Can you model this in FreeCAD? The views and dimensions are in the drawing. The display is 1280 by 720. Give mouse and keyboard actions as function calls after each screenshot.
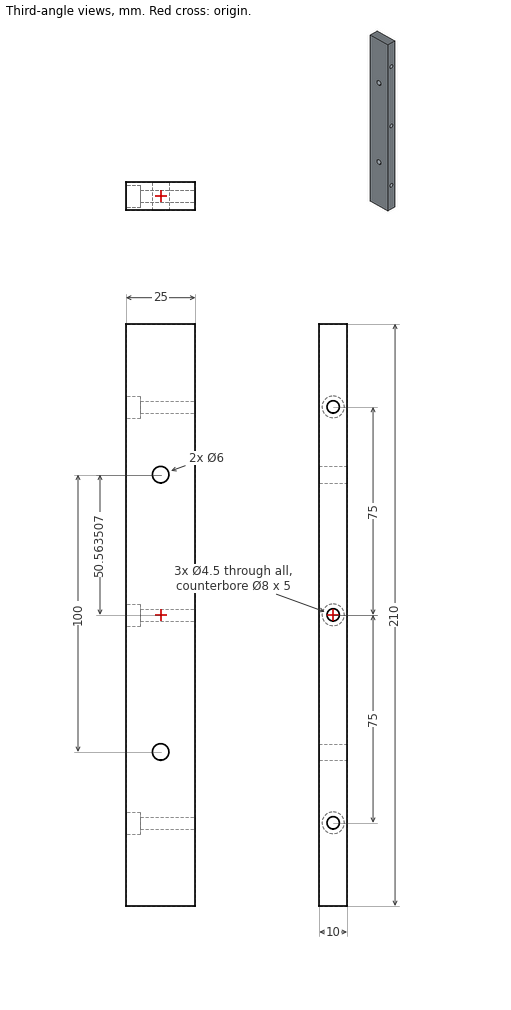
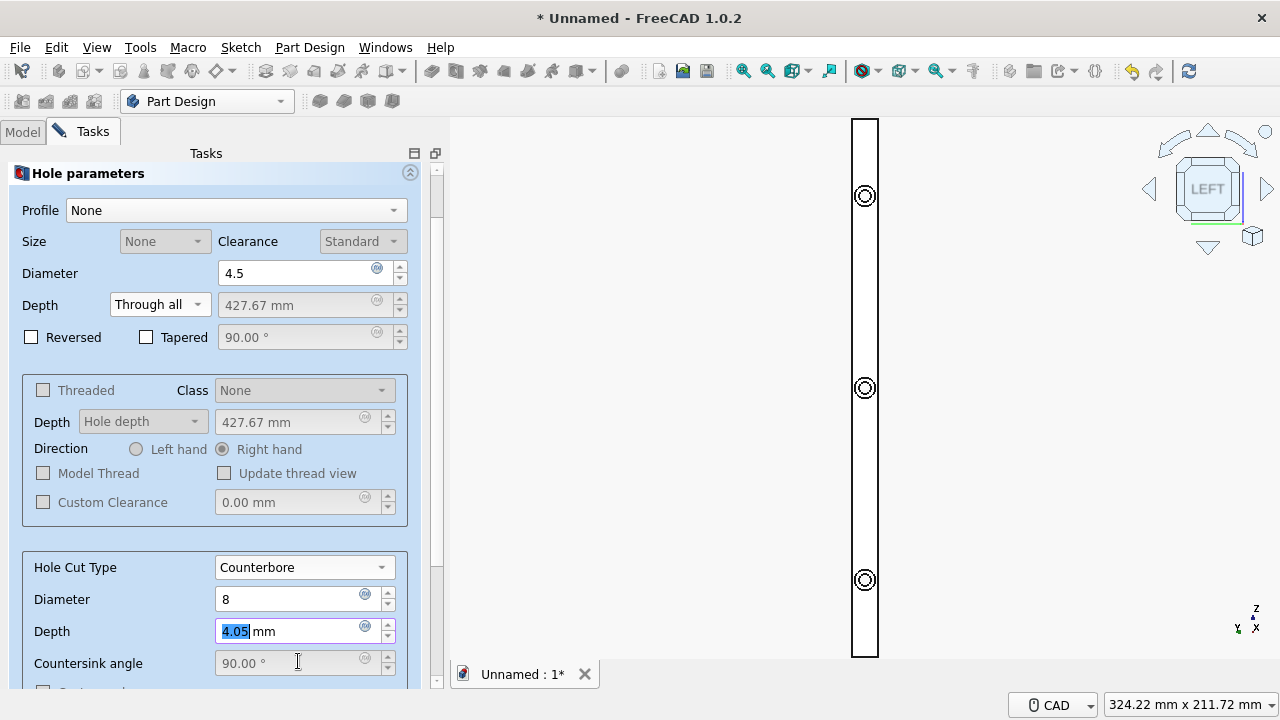
text(5)
key(Tab)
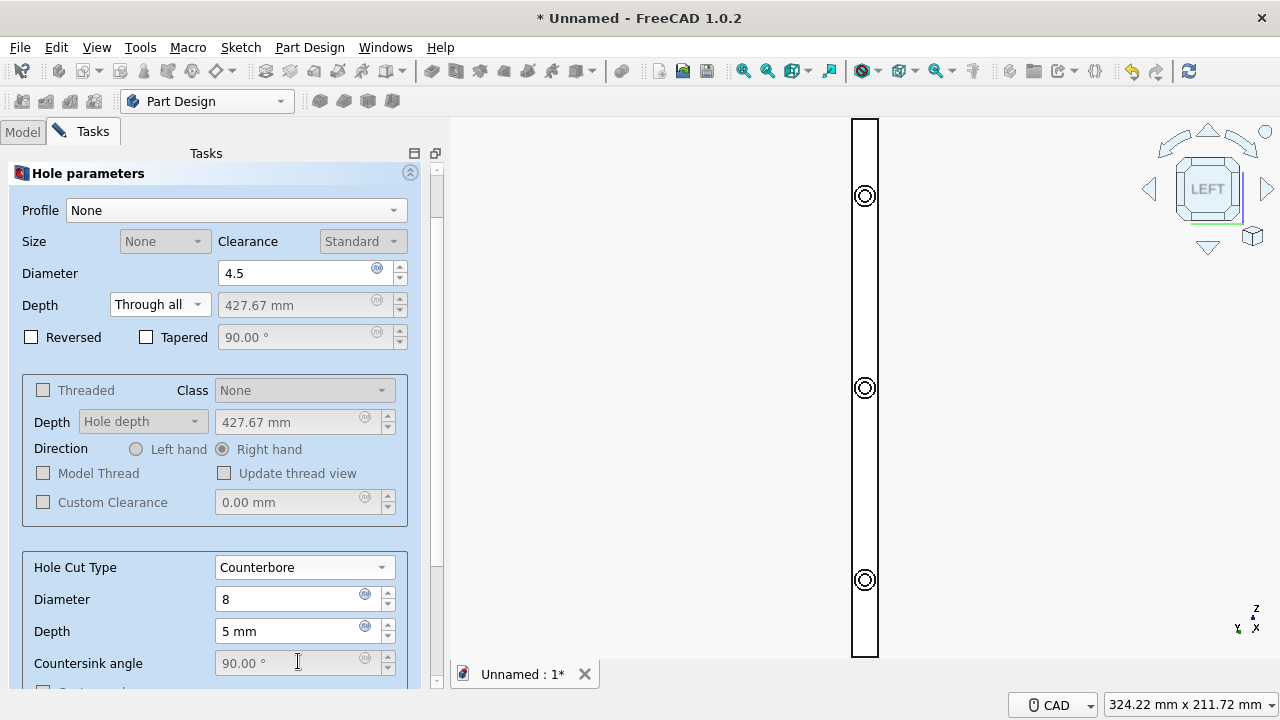
scroll(437, 426, up, 2)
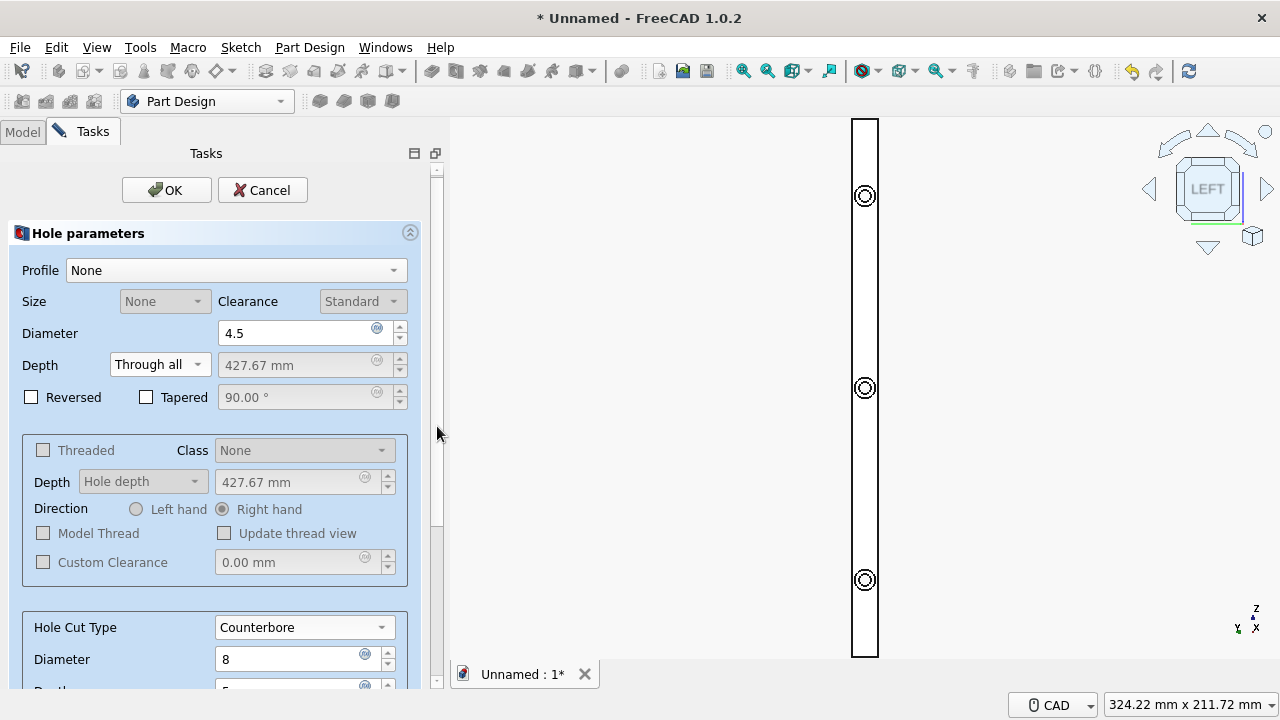
click(167, 192)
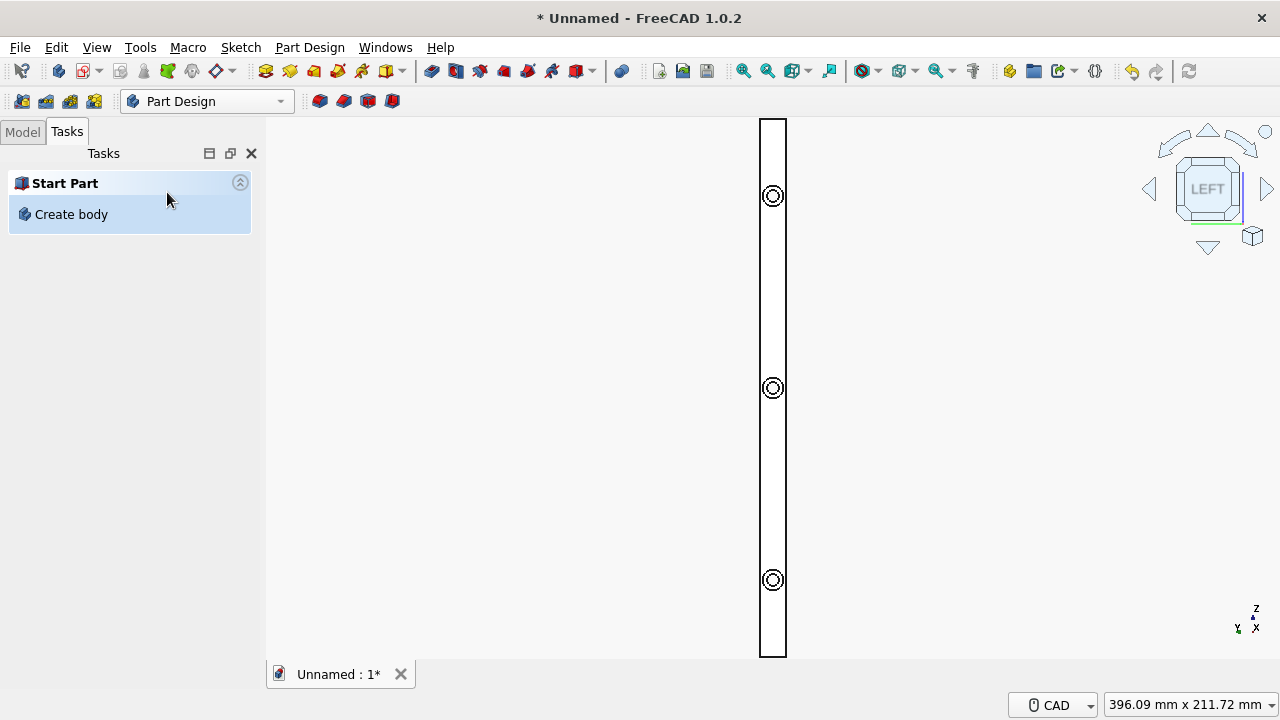
key(0)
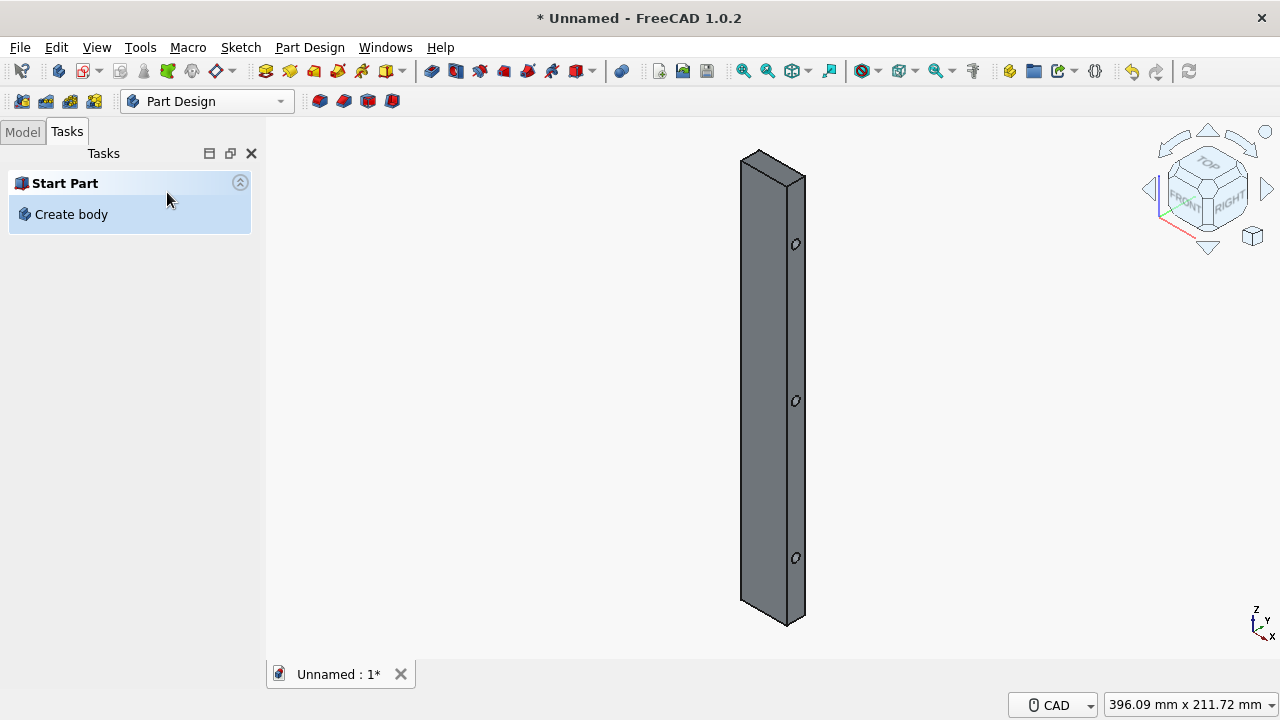
click(764, 580)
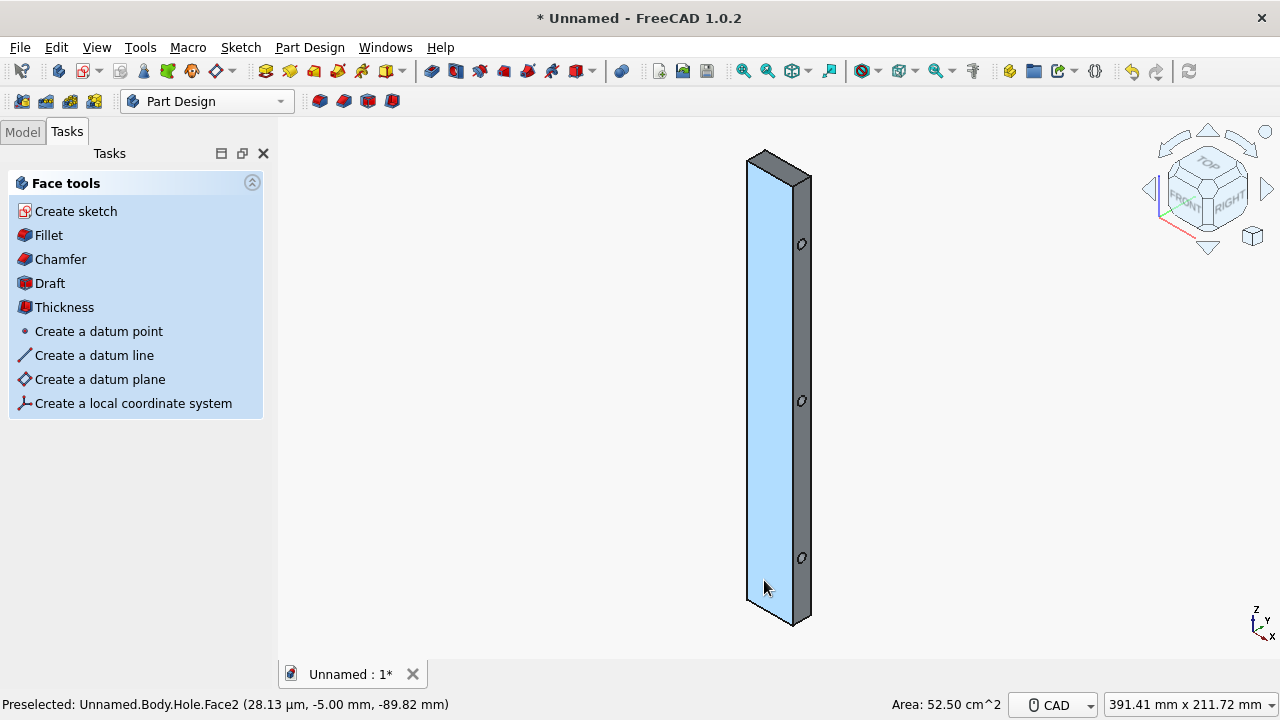
click(84, 72)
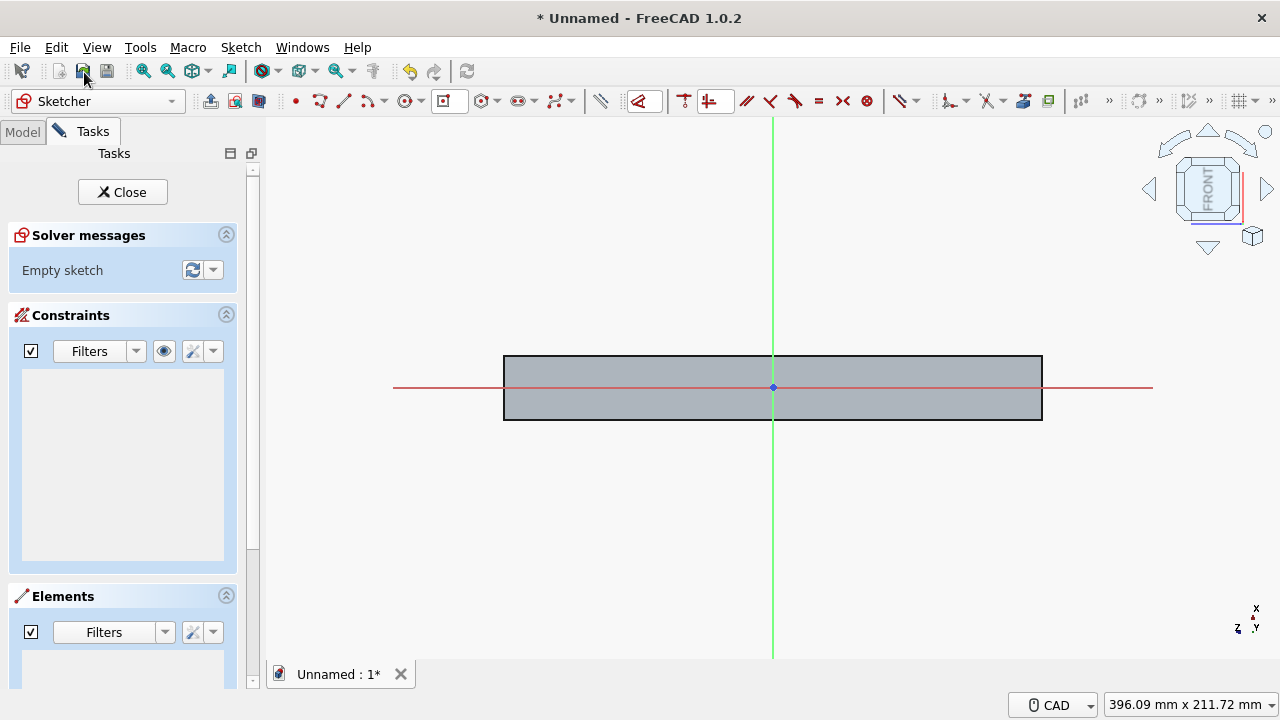
scroll(826, 388, up, 4)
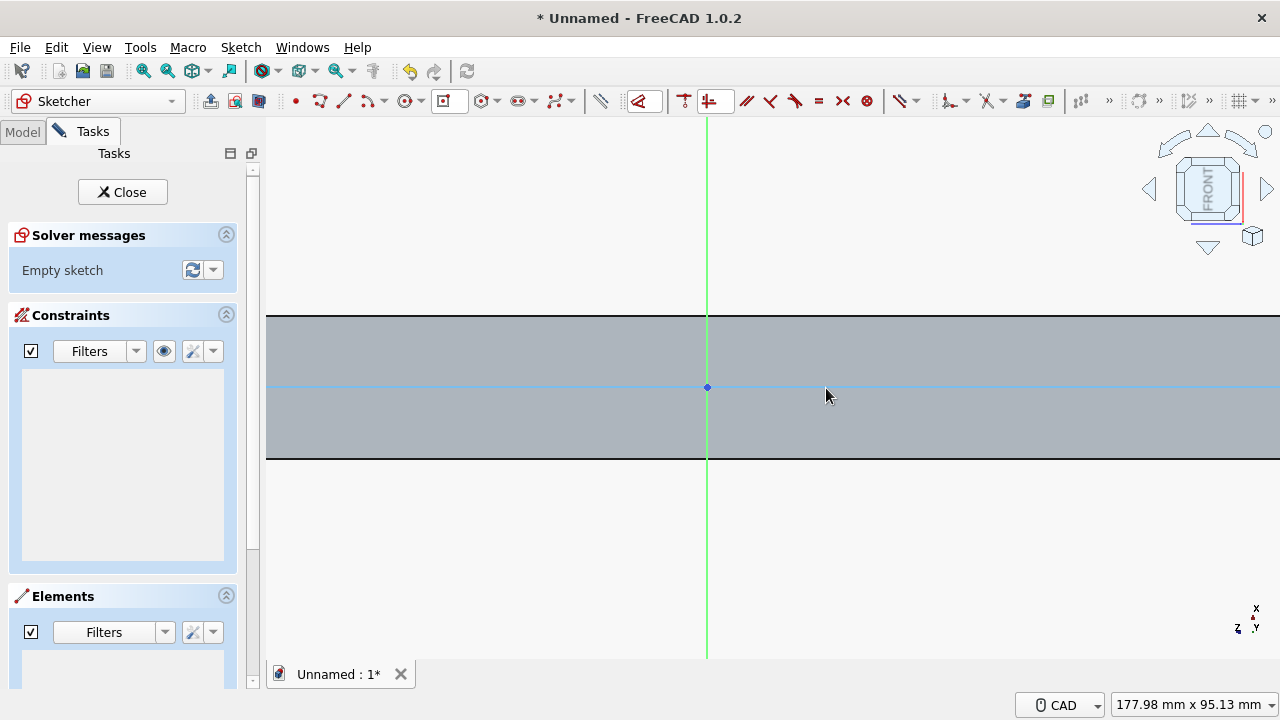
click(406, 102)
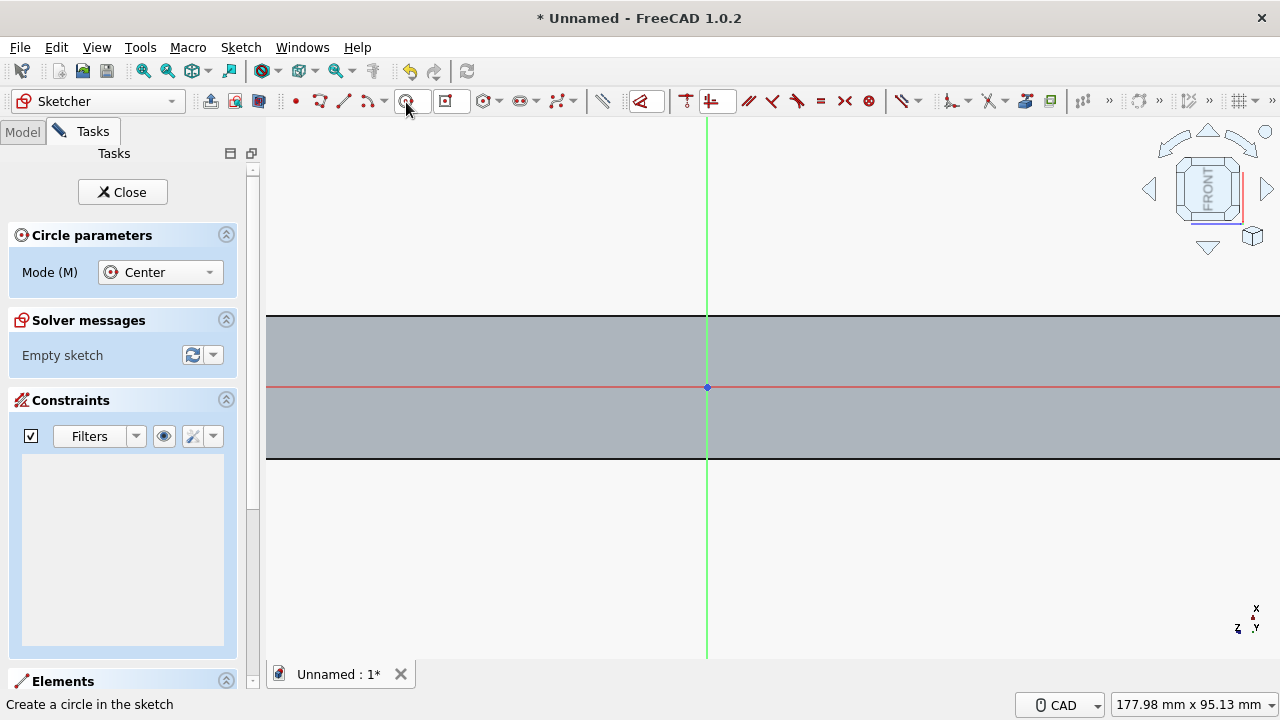
scroll(419, 387, up, 2)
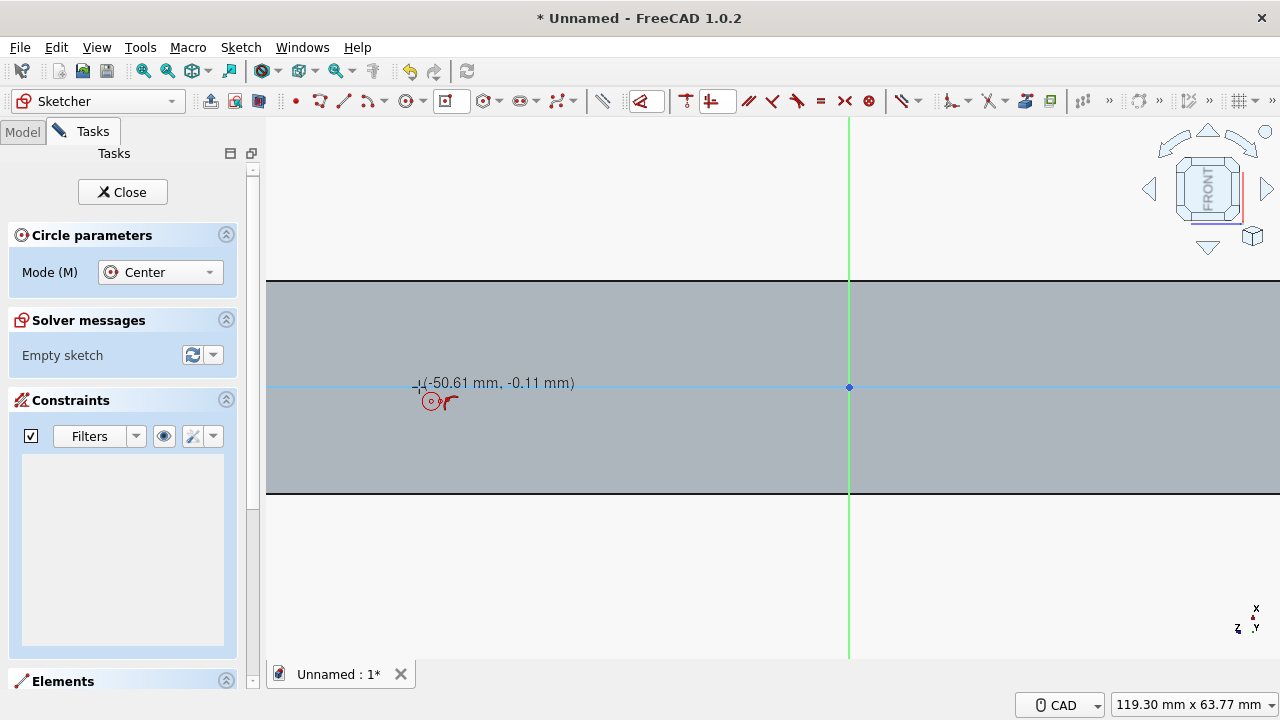
click(419, 387)
move(437, 369)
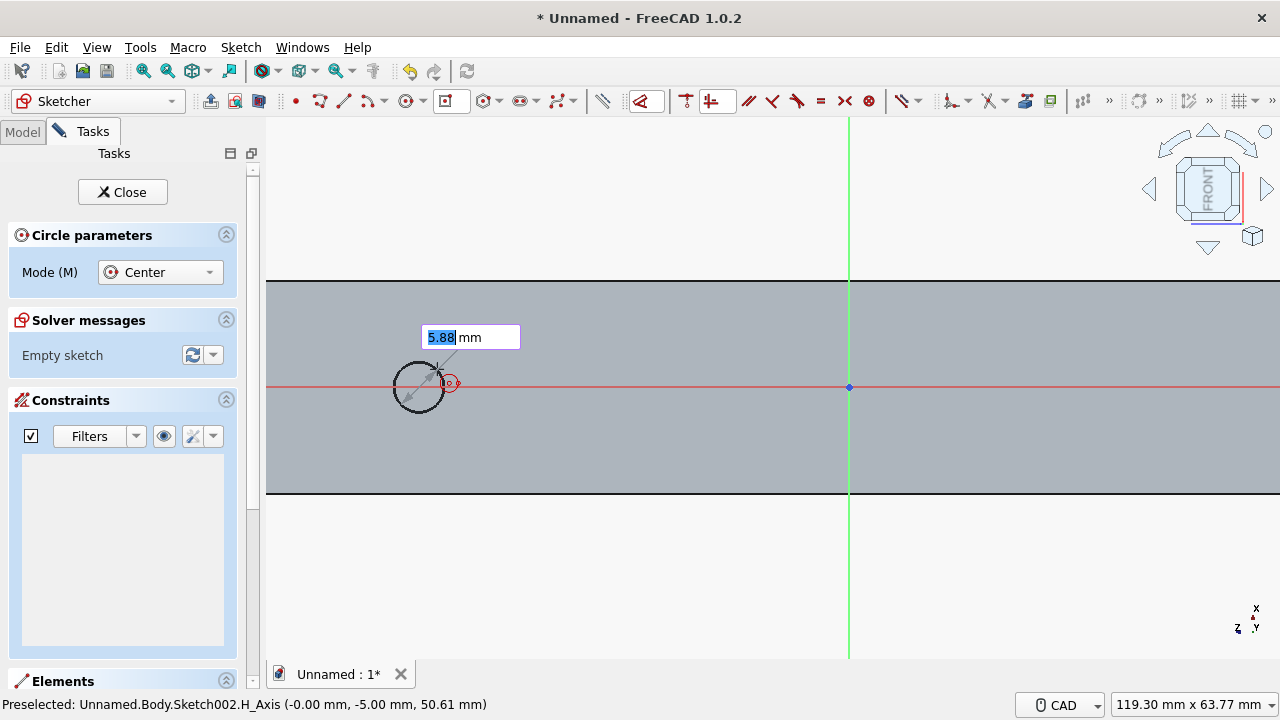
text(6)
key(Return)